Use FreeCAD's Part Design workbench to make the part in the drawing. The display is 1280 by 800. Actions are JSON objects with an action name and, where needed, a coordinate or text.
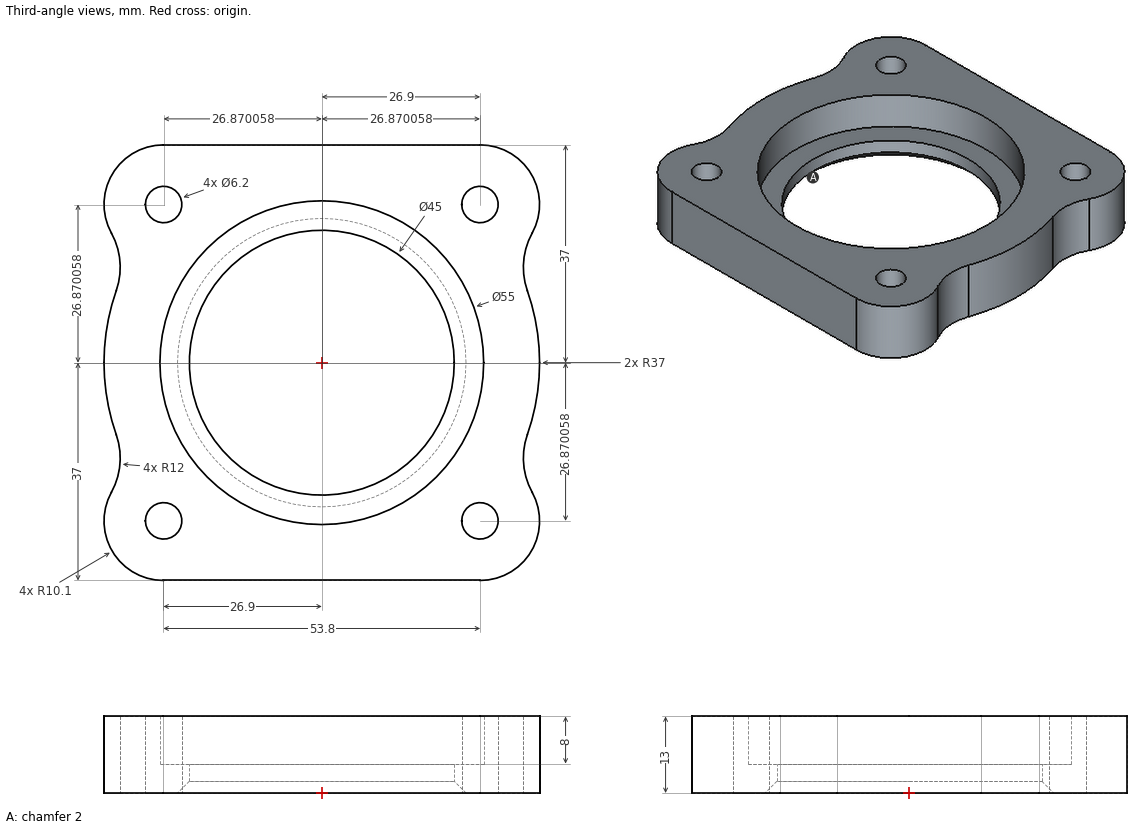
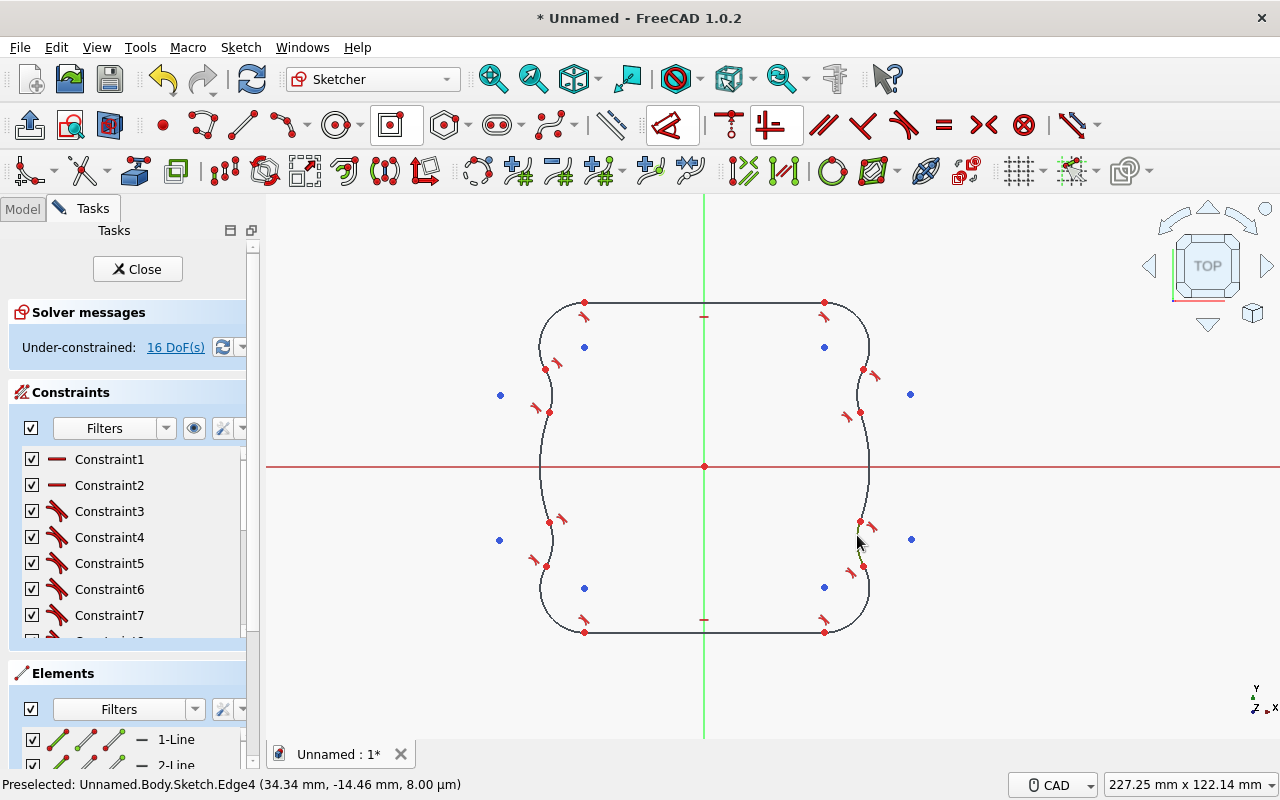
{"action": "left_click", "coordinate": [859, 381]}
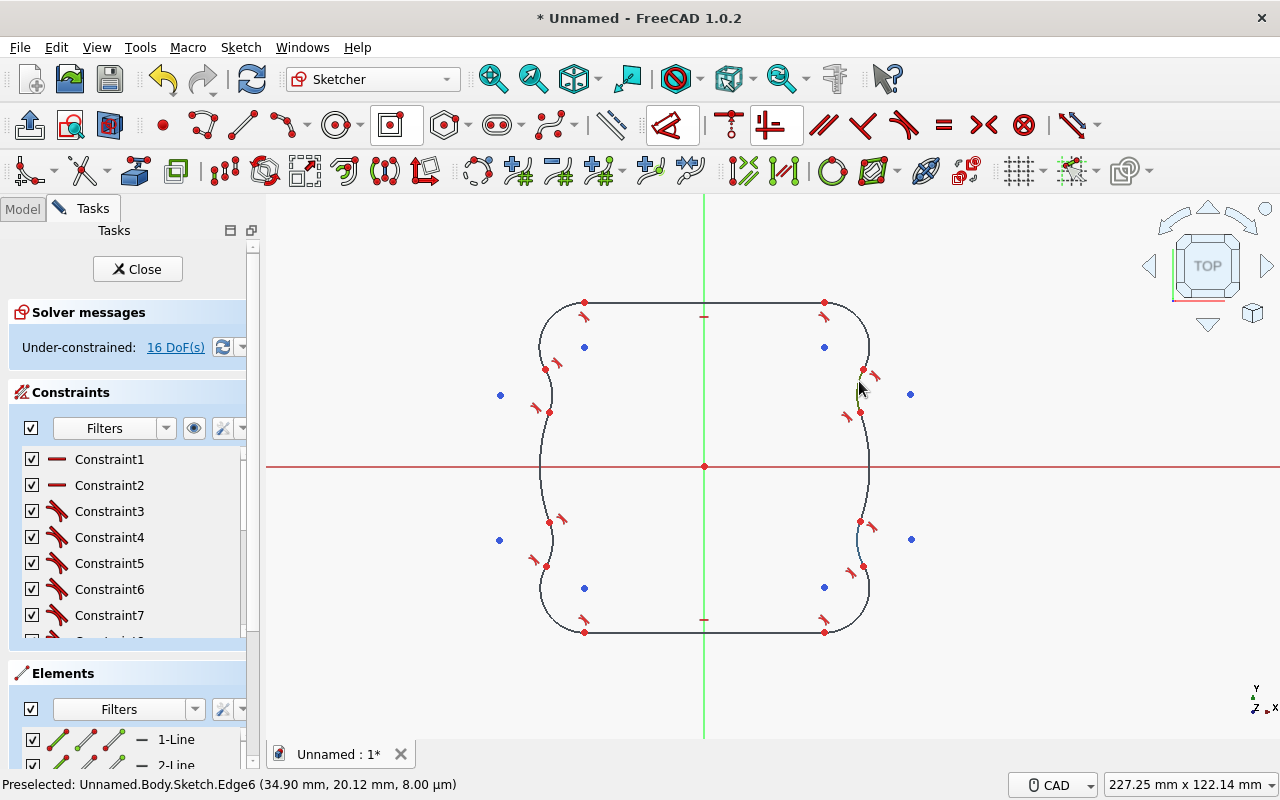
{"action": "left_click", "coordinate": [552, 400]}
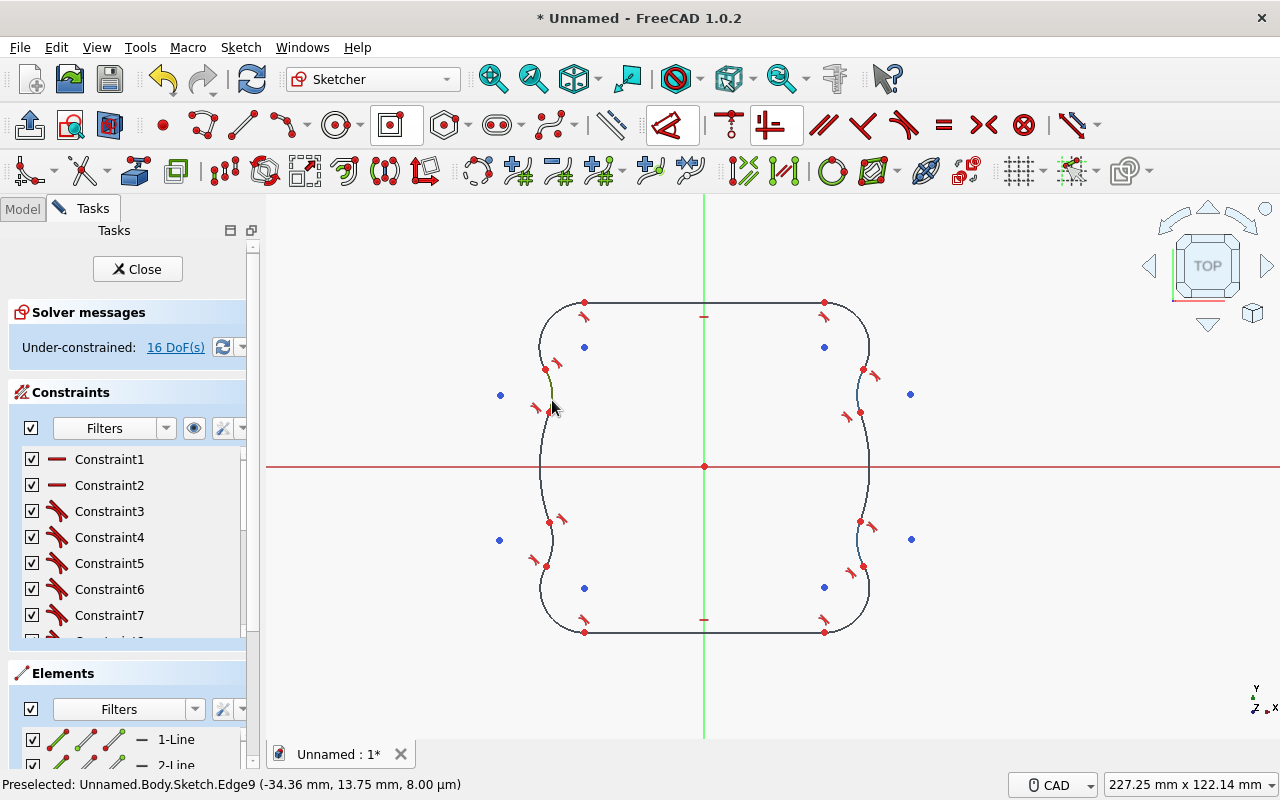
{"action": "left_click", "coordinate": [551, 554]}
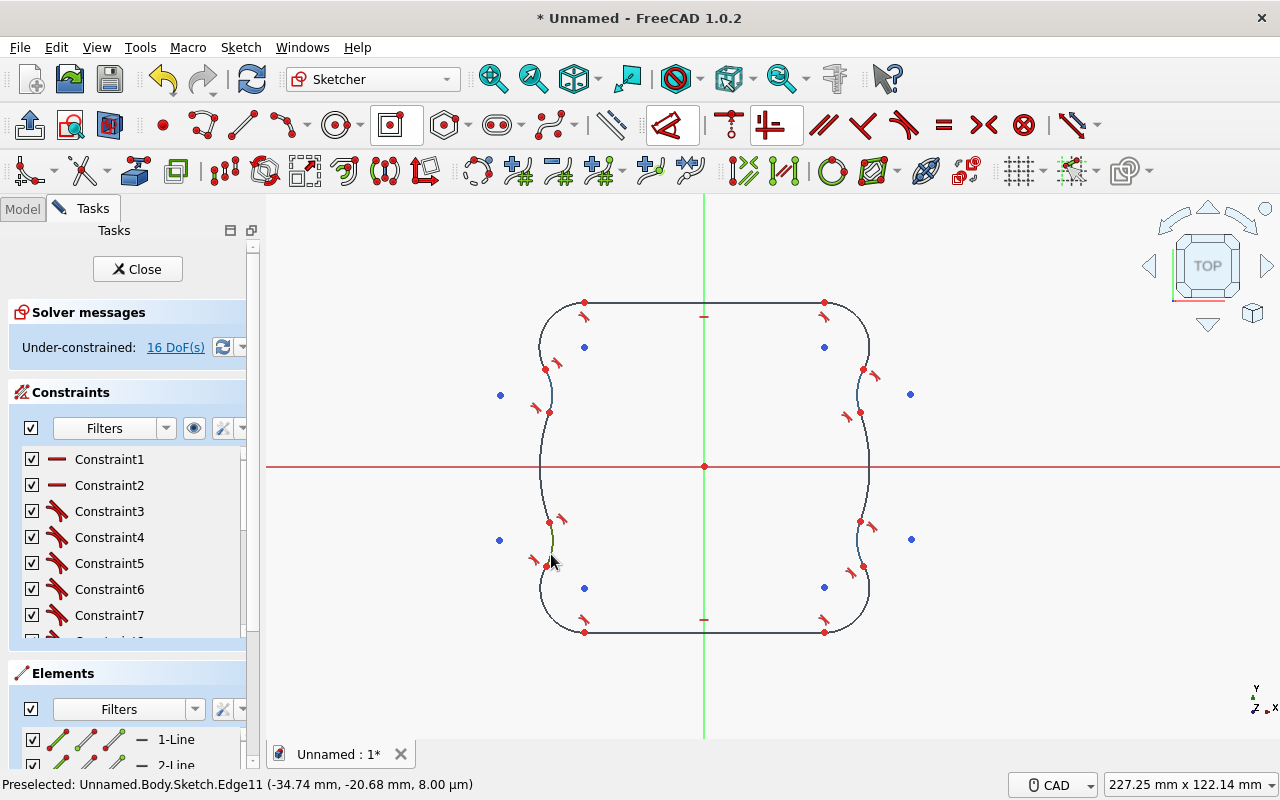
{"action": "left_click", "coordinate": [944, 126]}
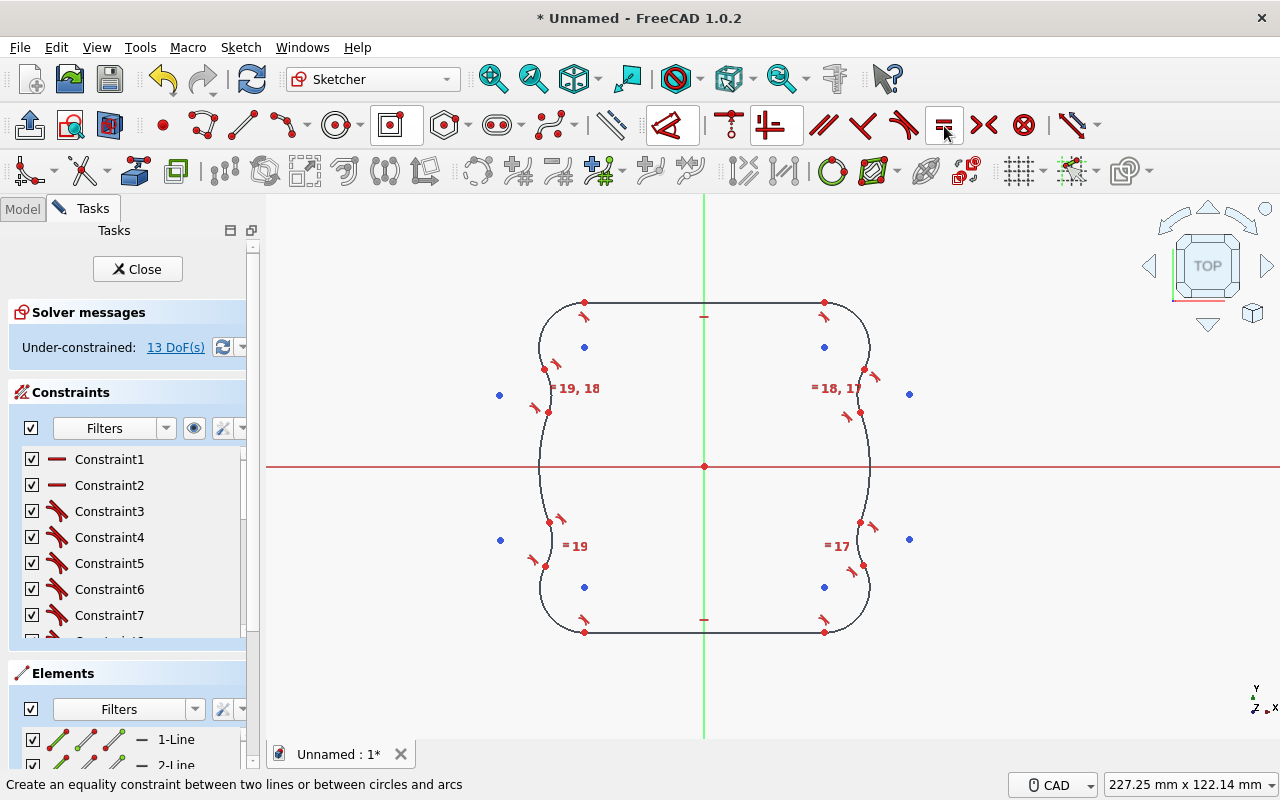
{"action": "left_click", "coordinate": [851, 624]}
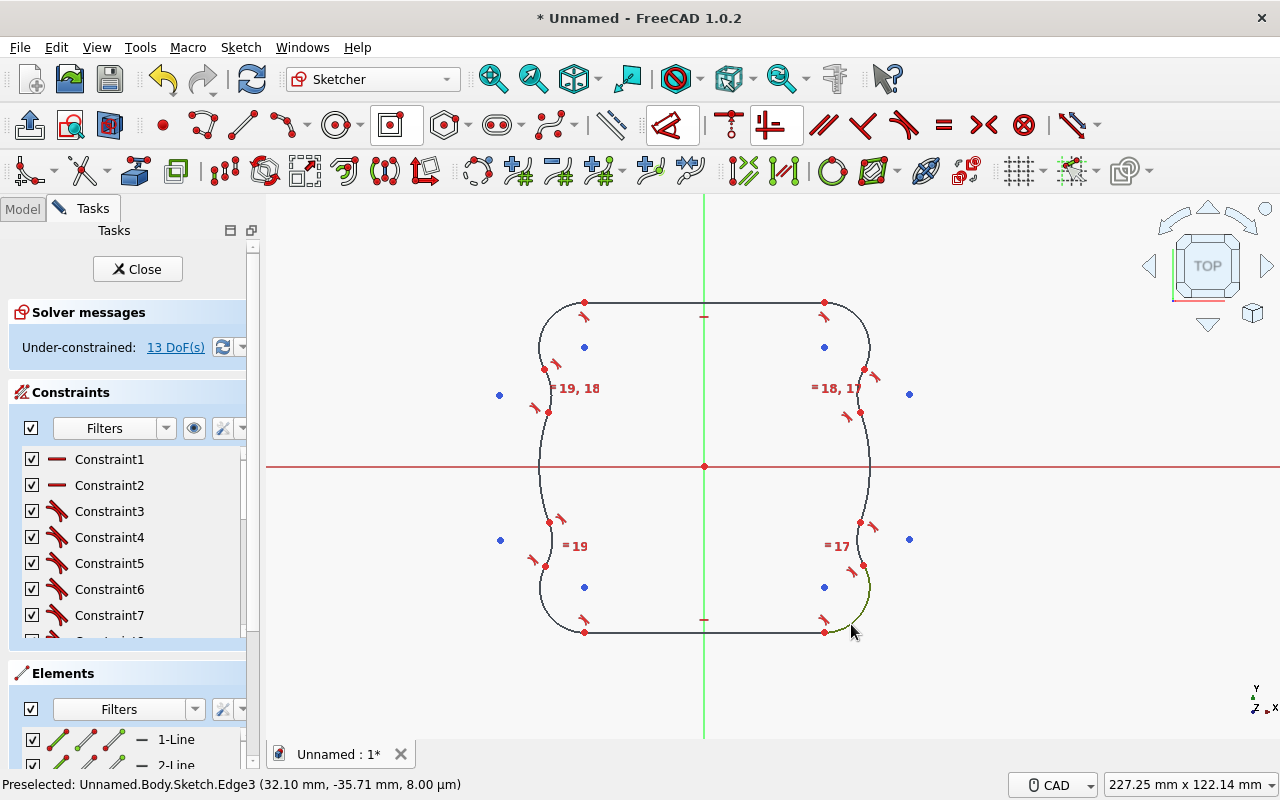
{"action": "left_click", "coordinate": [869, 342]}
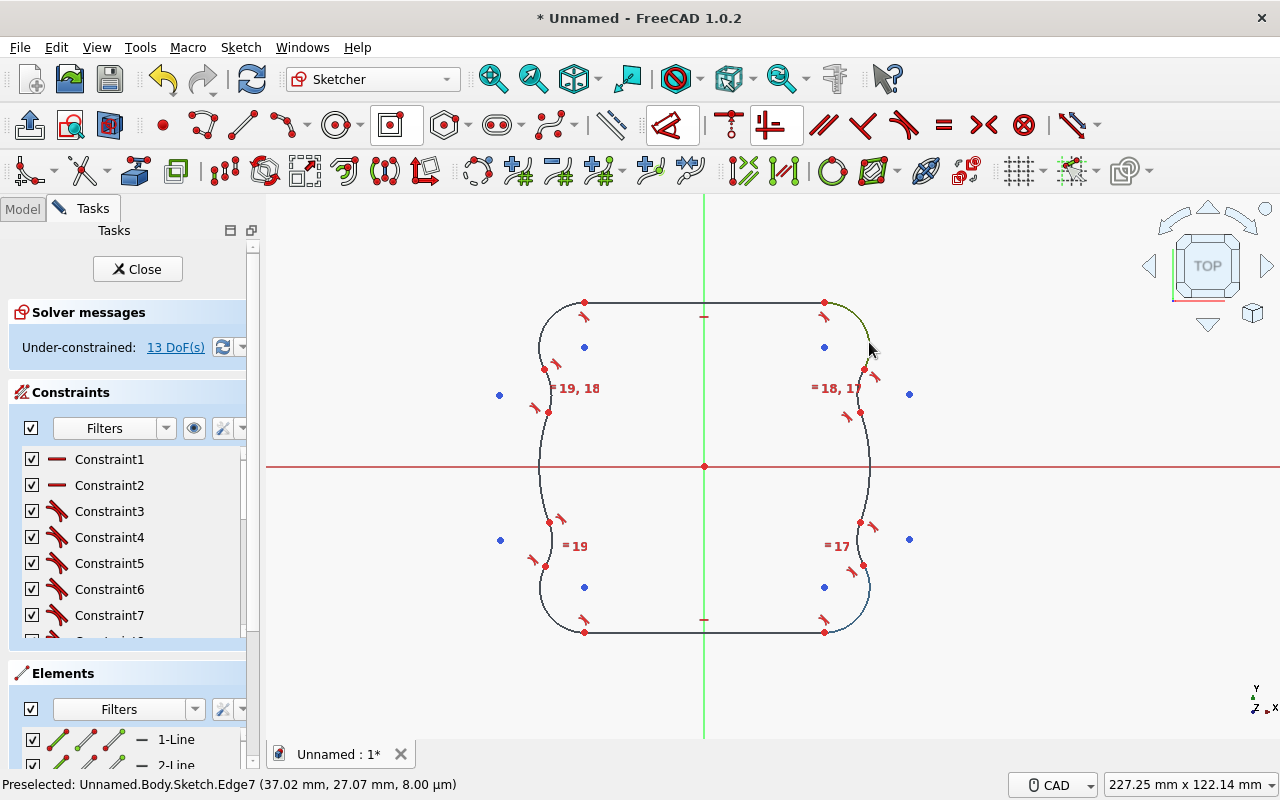
{"action": "left_click", "coordinate": [558, 311]}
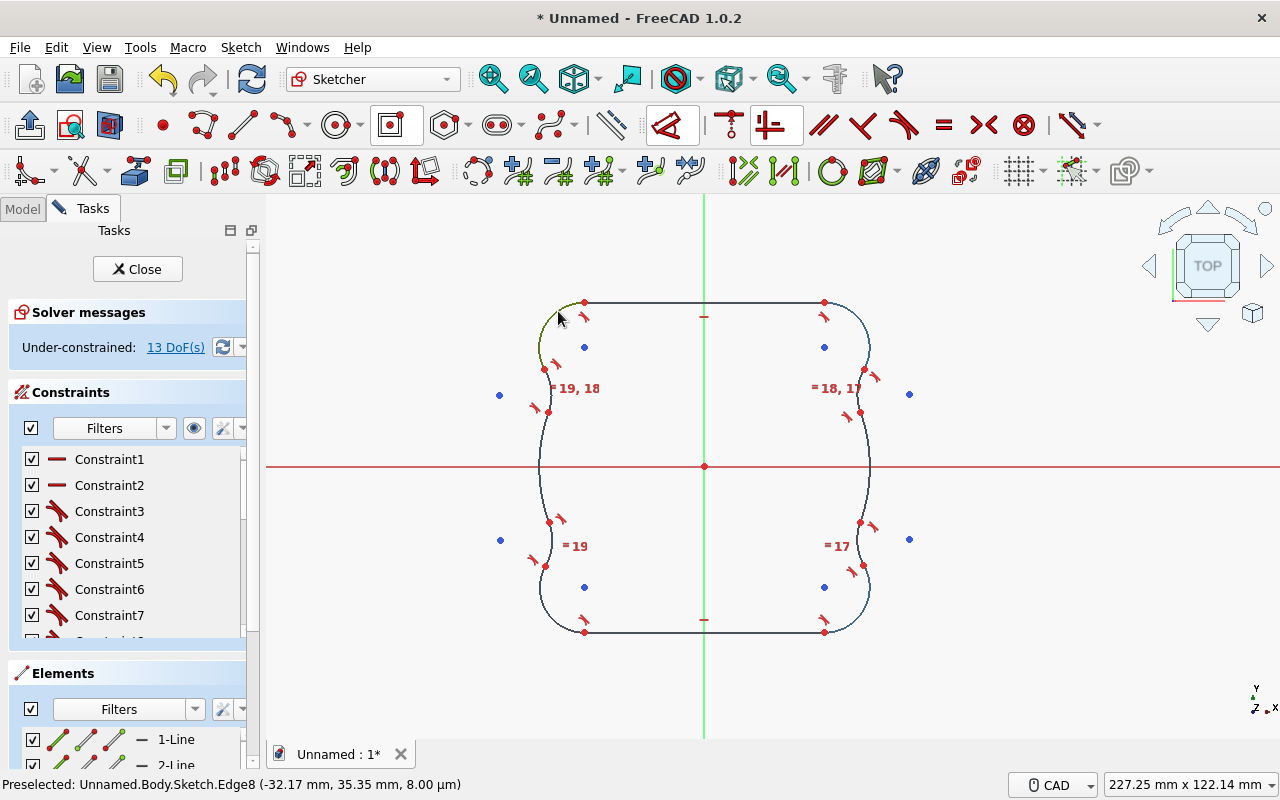
{"action": "left_click", "coordinate": [540, 593]}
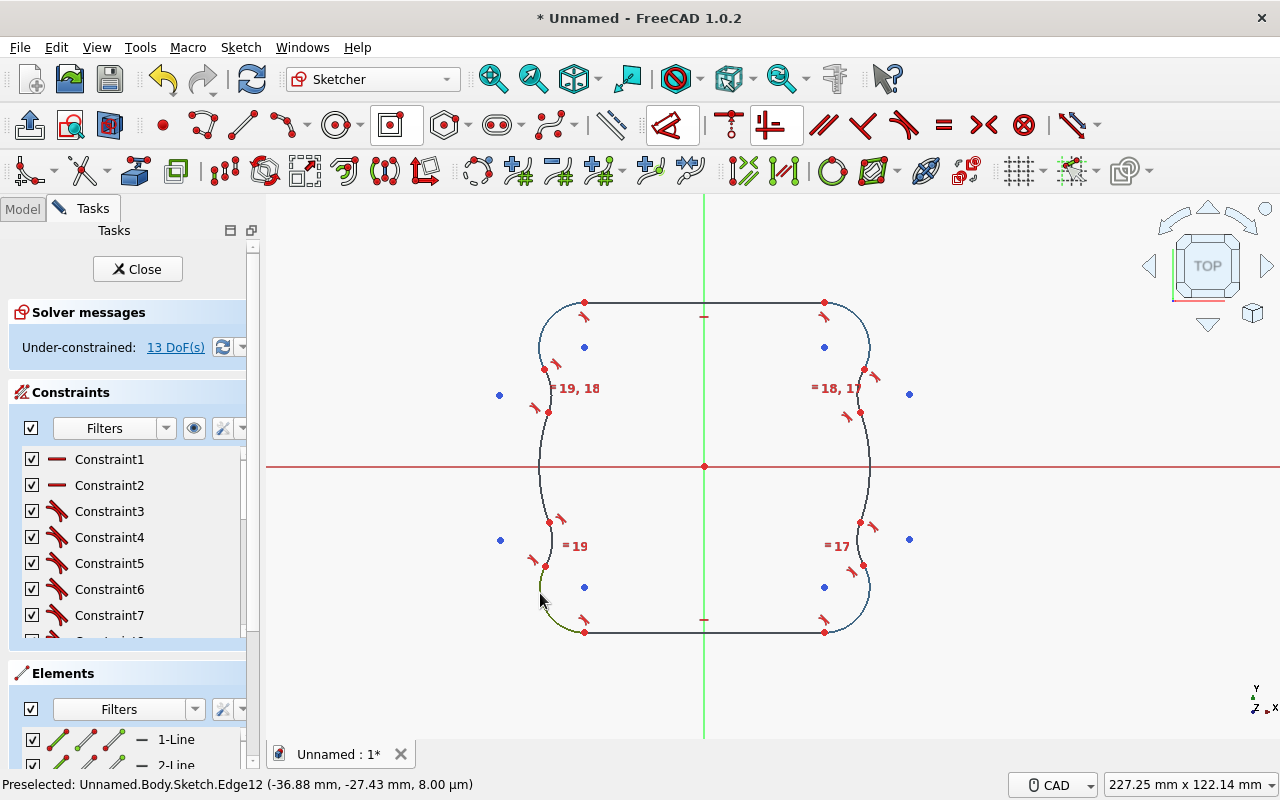
{"action": "key", "text": "e"}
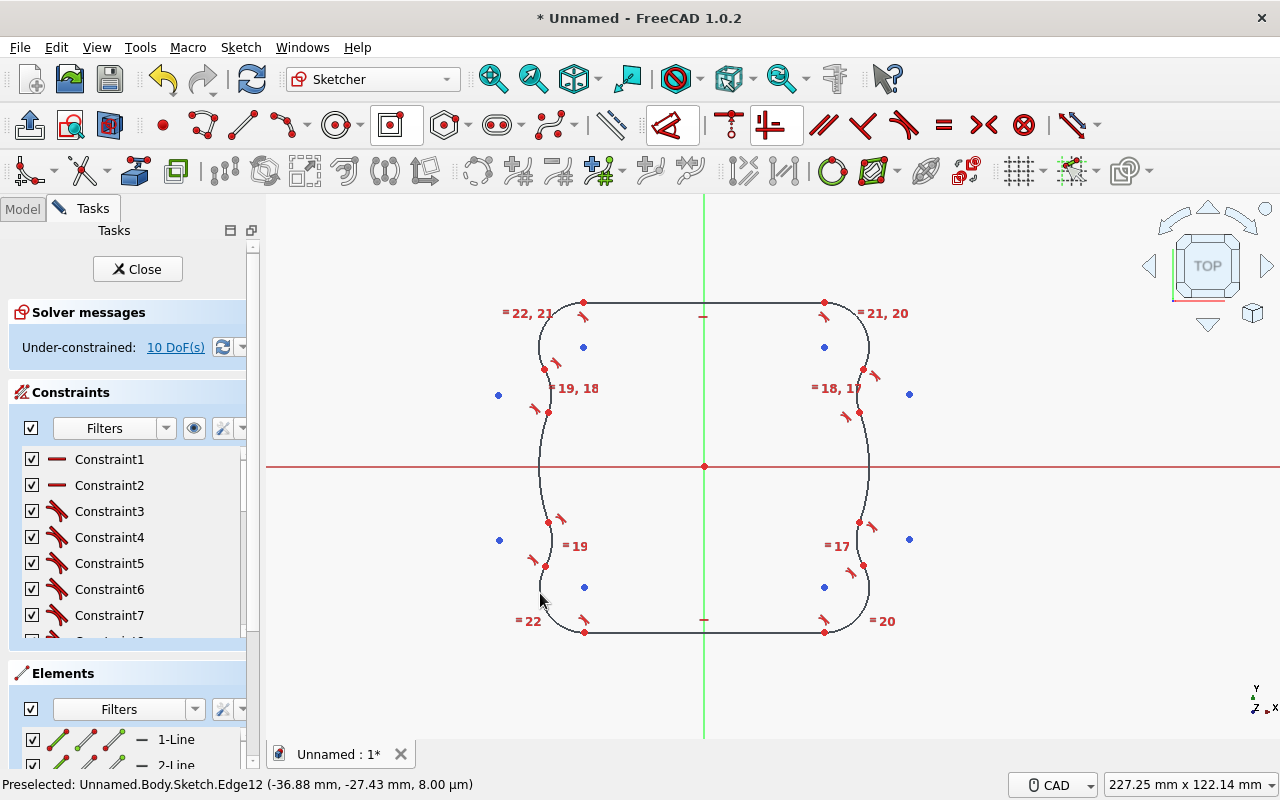
{"action": "left_click", "coordinate": [868, 490]}